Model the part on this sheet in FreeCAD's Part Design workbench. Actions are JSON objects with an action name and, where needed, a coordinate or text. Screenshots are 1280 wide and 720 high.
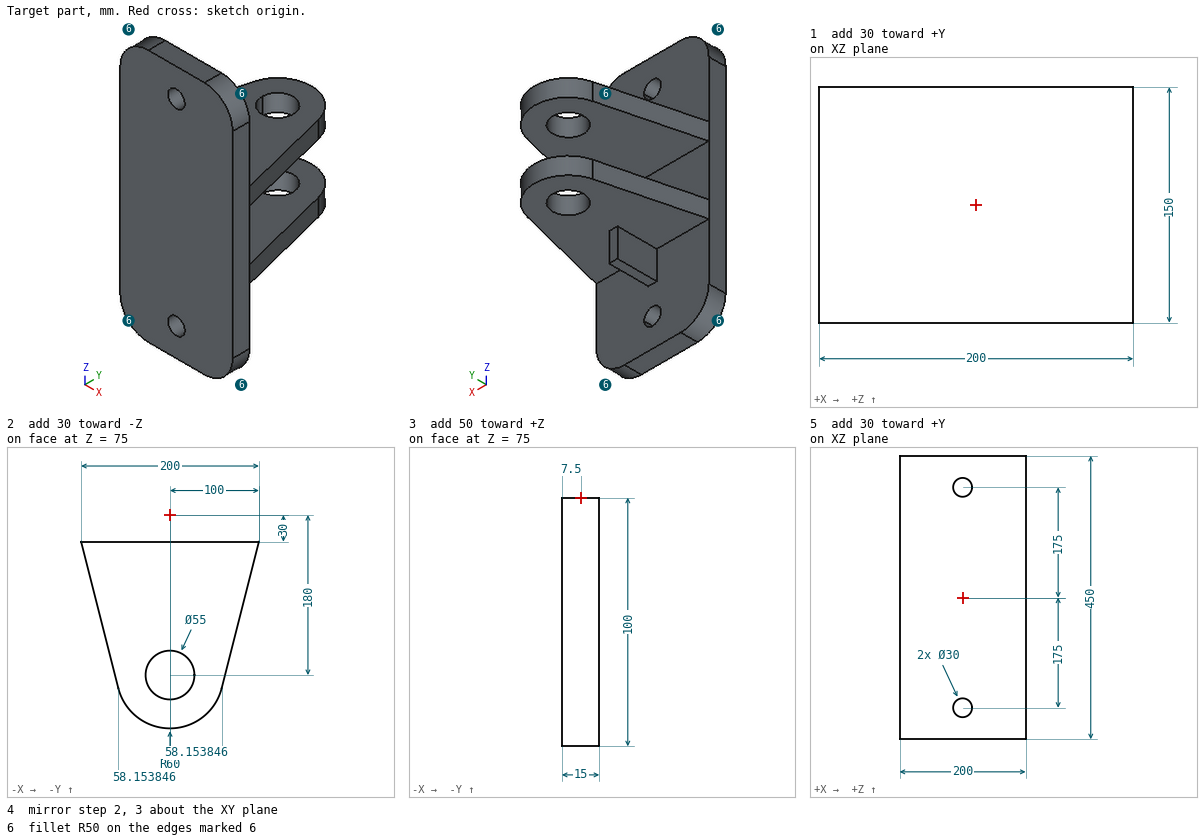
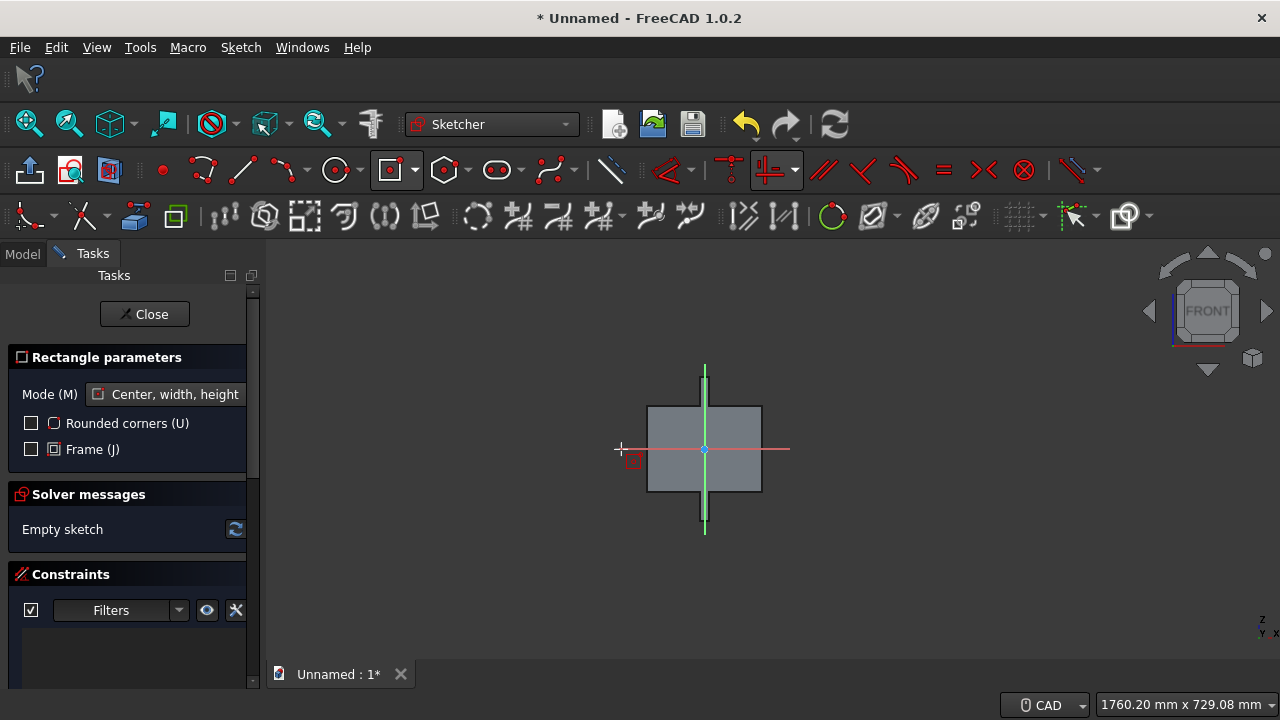
{"action": "left_click", "coordinate": [705, 449]}
{"action": "mouse_move", "coordinate": [762, 320]}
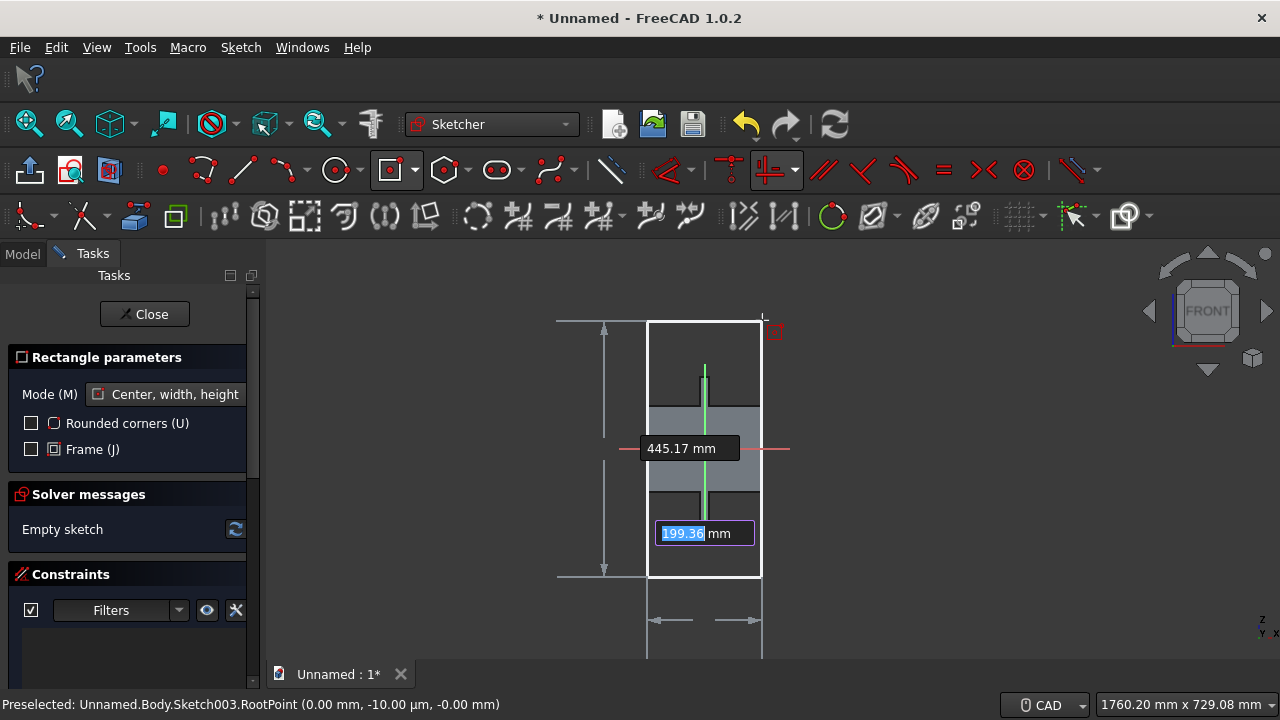
{"action": "type", "text": "200"}
{"action": "key", "text": "Tab"}
{"action": "type", "text": "450"}
{"action": "key", "text": "Return"}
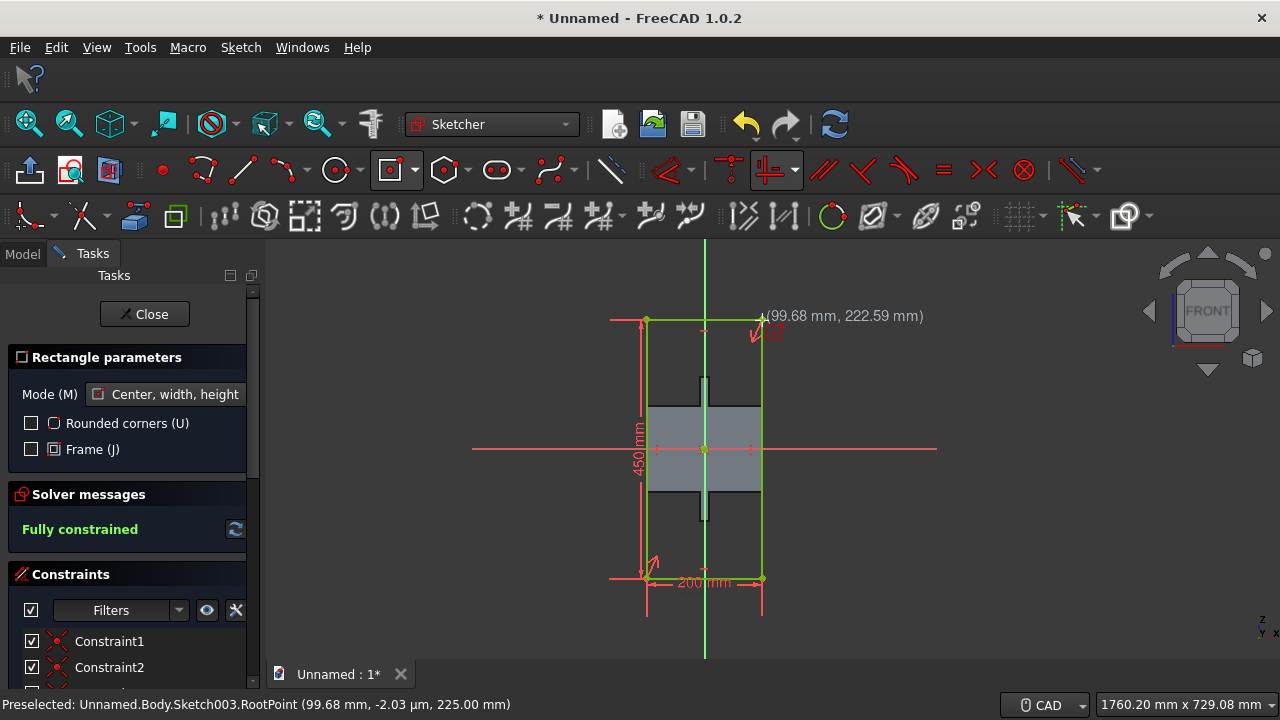
{"action": "key", "text": "g c"}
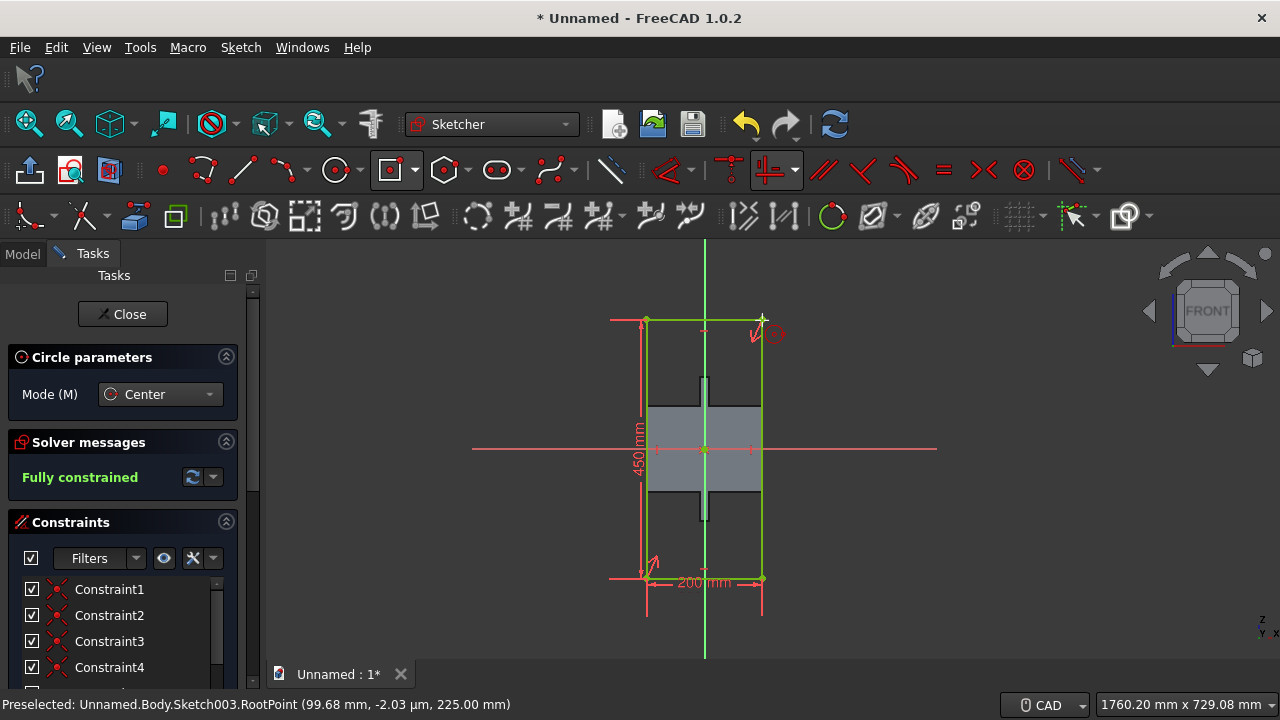
{"action": "scroll", "coordinate": [705, 550], "scroll_direction": "up", "scroll_amount": 5}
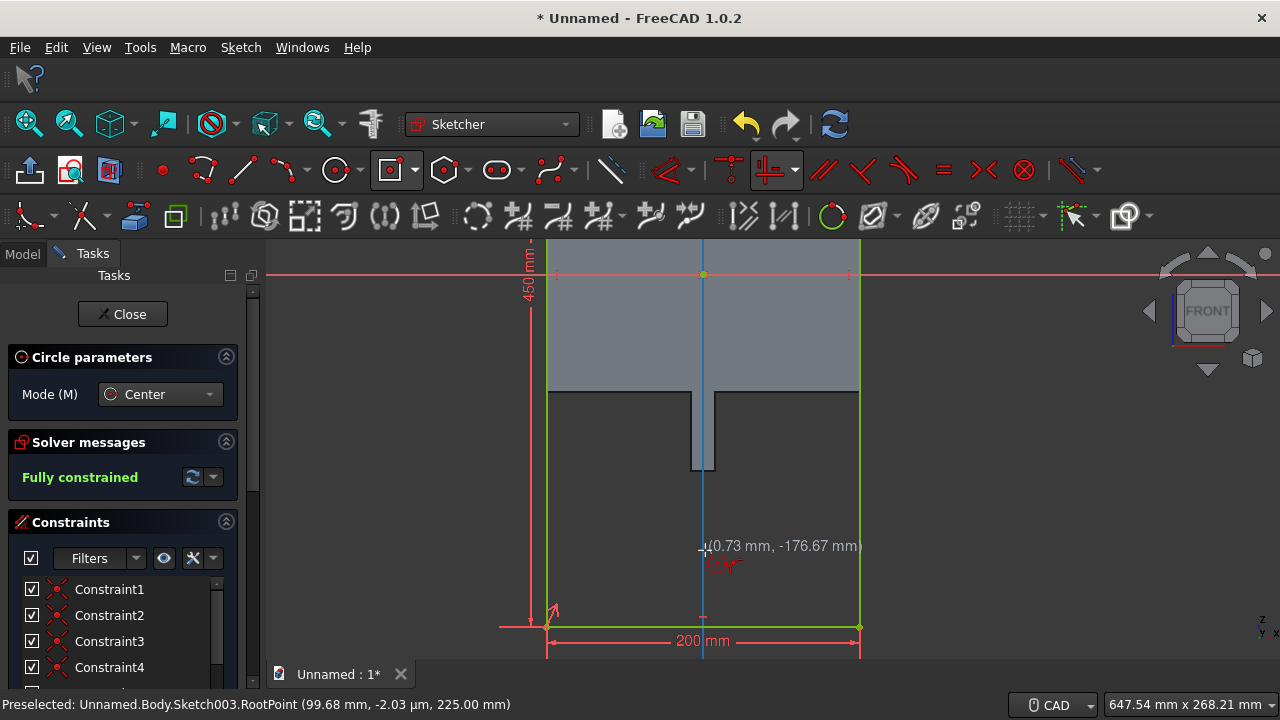
{"action": "left_click", "coordinate": [703, 549]}
{"action": "mouse_move", "coordinate": [720, 532]}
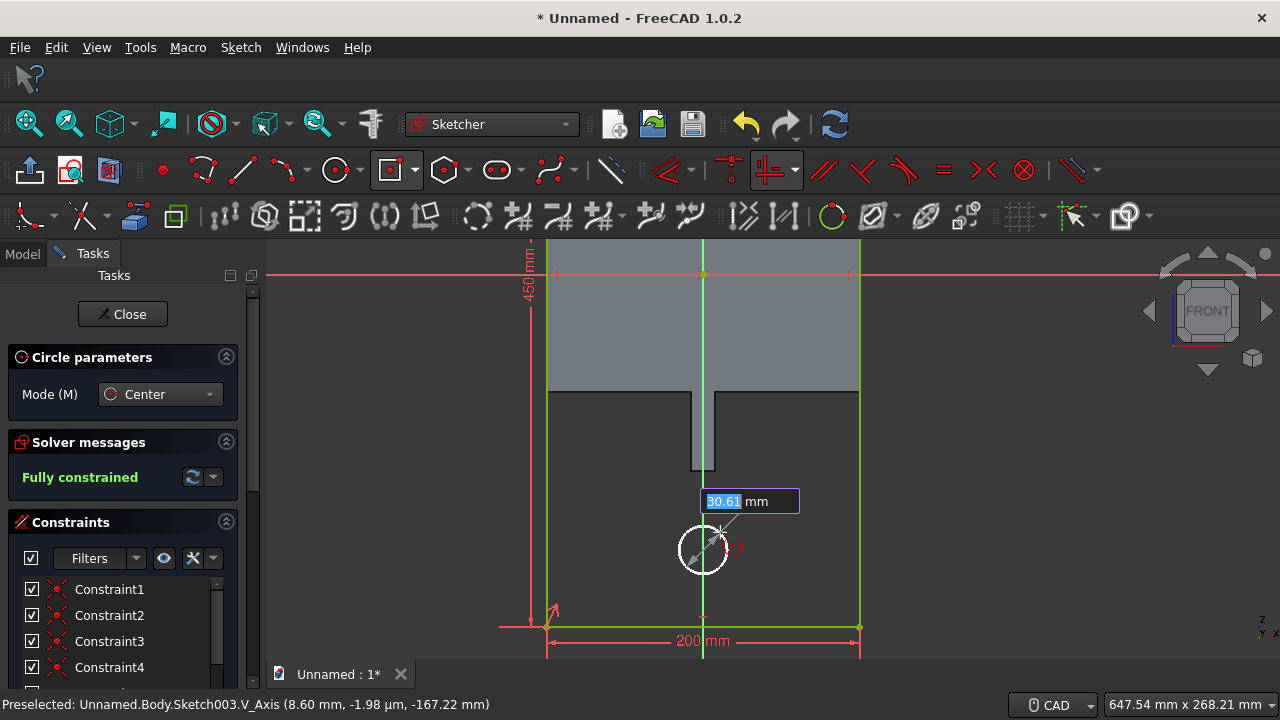
{"action": "type", "text": "30"}
{"action": "key", "text": "Return"}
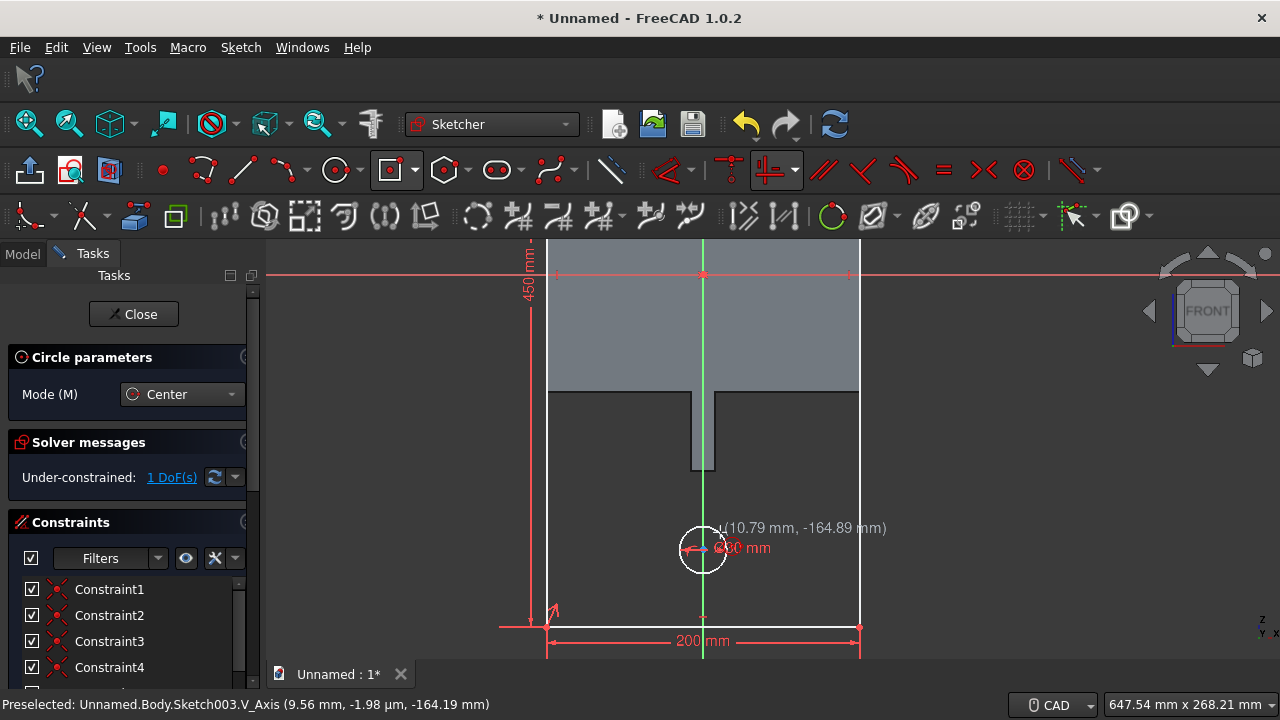
{"action": "scroll", "coordinate": [705, 550], "scroll_direction": "down", "scroll_amount": 5}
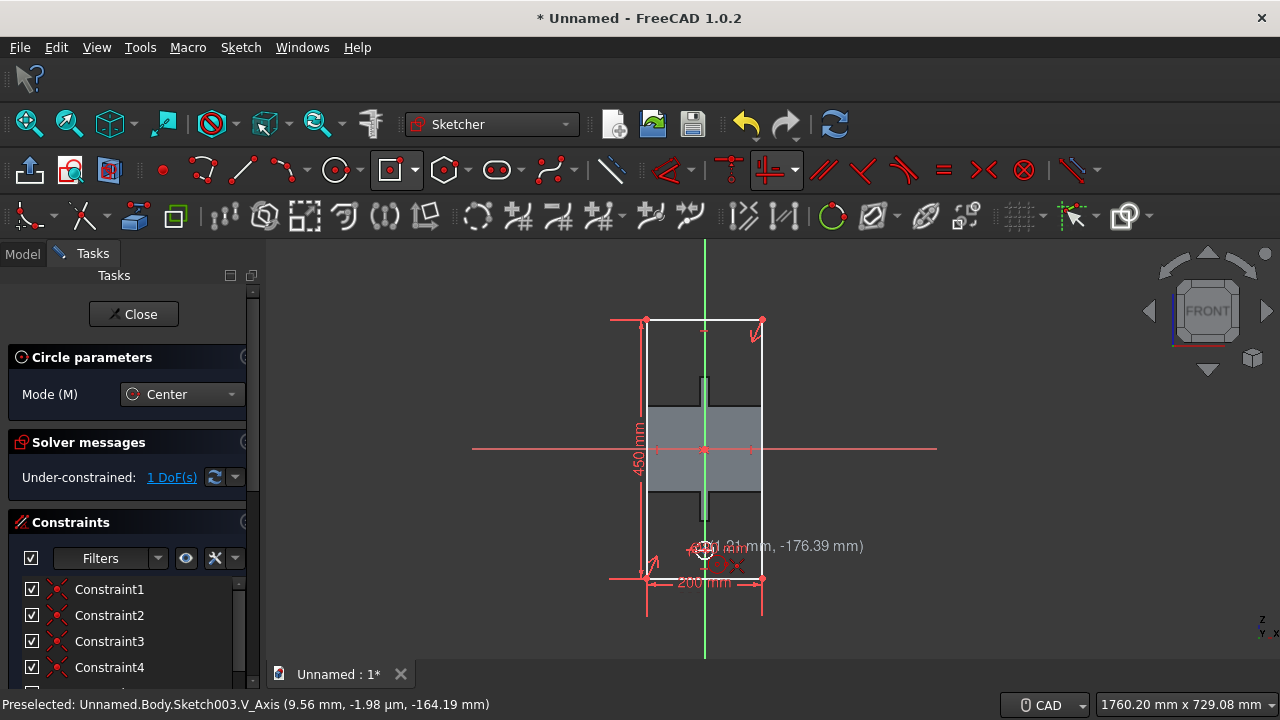
{"action": "scroll", "coordinate": [705, 348], "scroll_direction": "up", "scroll_amount": 5}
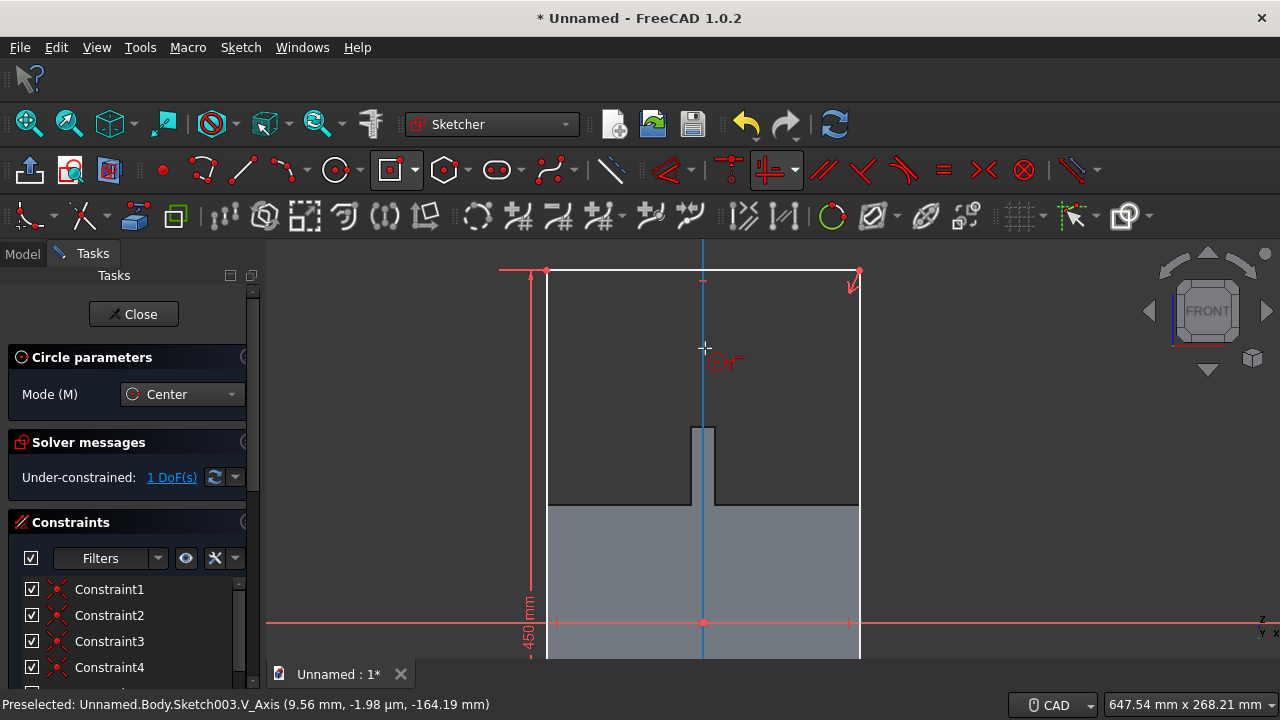
{"action": "left_click", "coordinate": [703, 349]}
{"action": "mouse_move", "coordinate": [720, 332]}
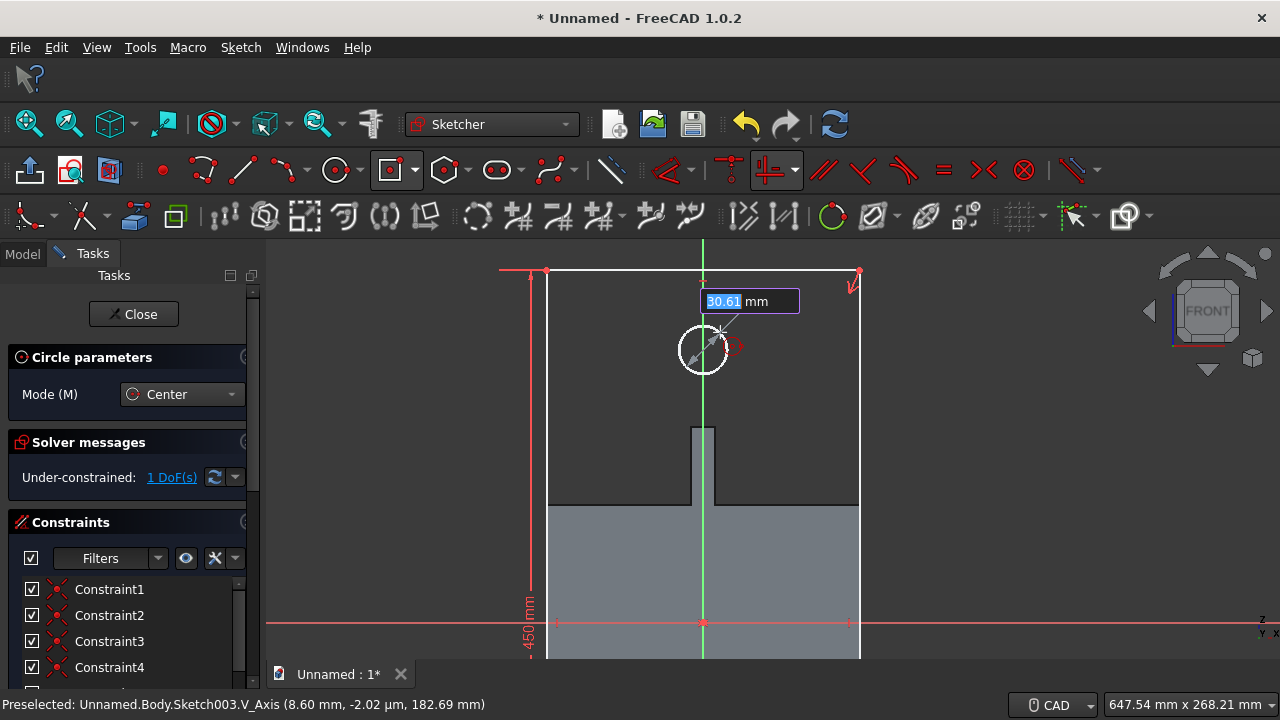
{"action": "type", "text": "30"}
{"action": "key", "text": "Return"}
{"action": "key", "text": "Escape"}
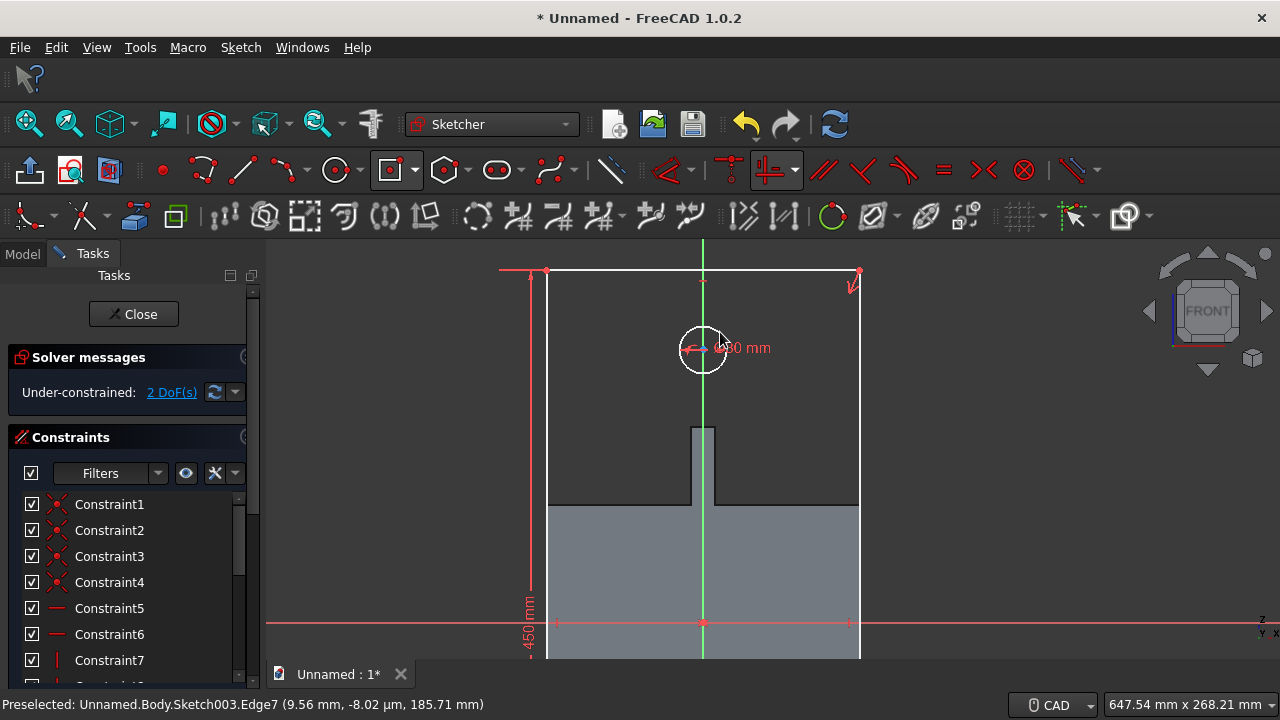
{"action": "key", "text": "d"}